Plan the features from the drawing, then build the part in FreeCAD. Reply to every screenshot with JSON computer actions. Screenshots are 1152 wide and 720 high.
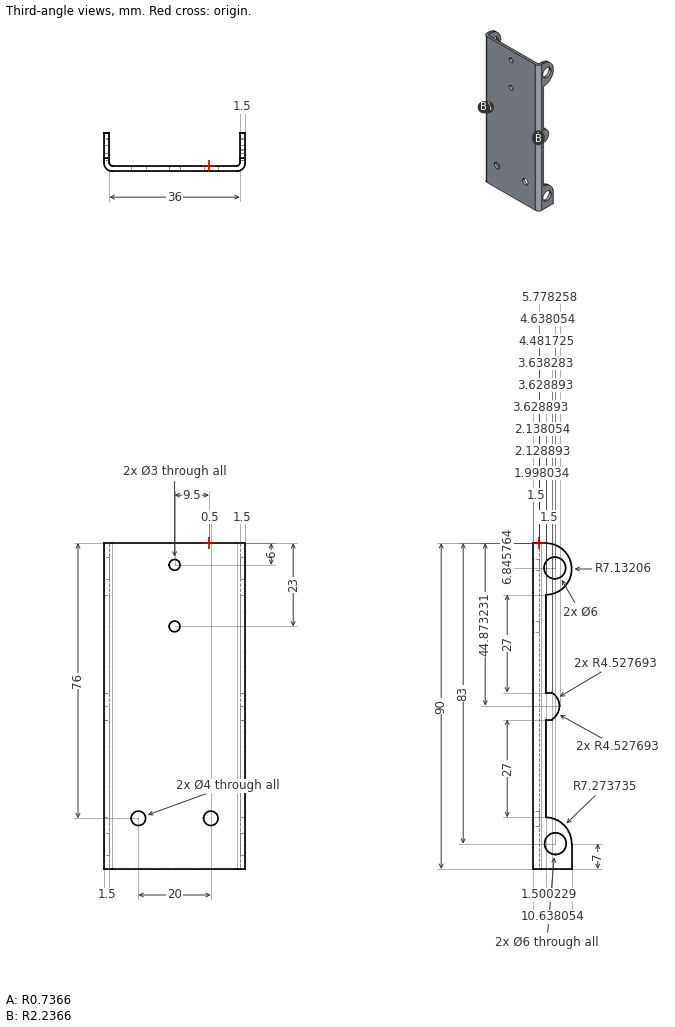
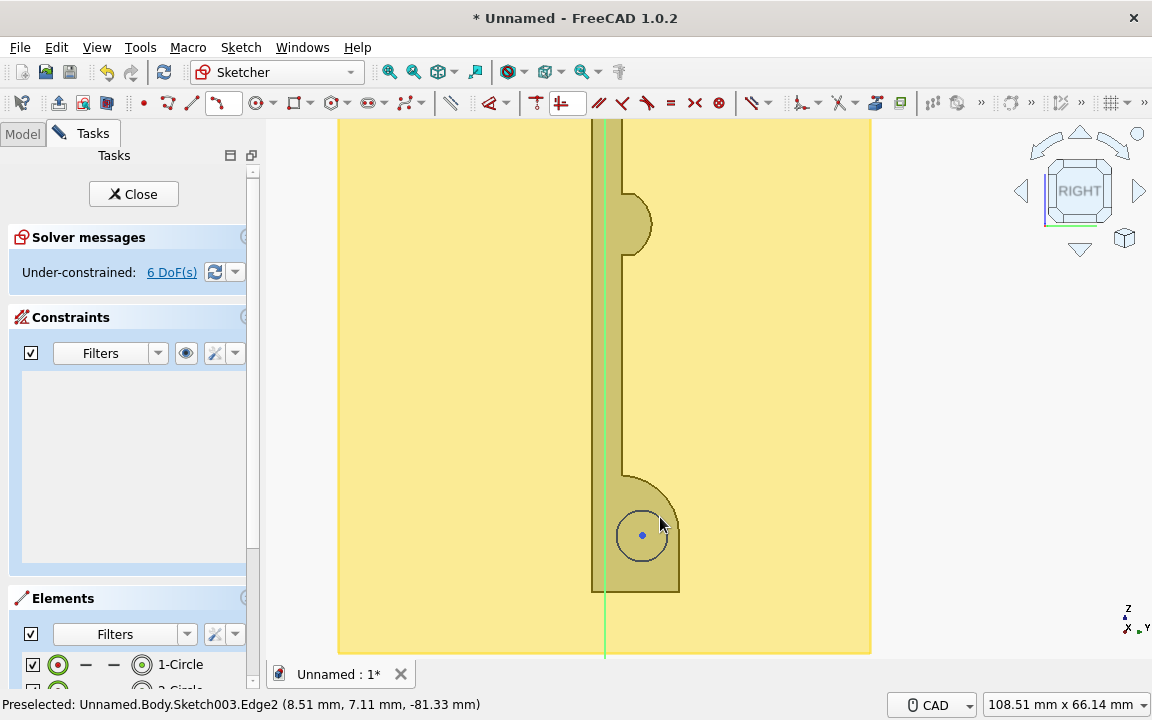
{"action": "scroll", "coordinate": [644, 537], "scroll_direction": "down", "scroll_amount": 4}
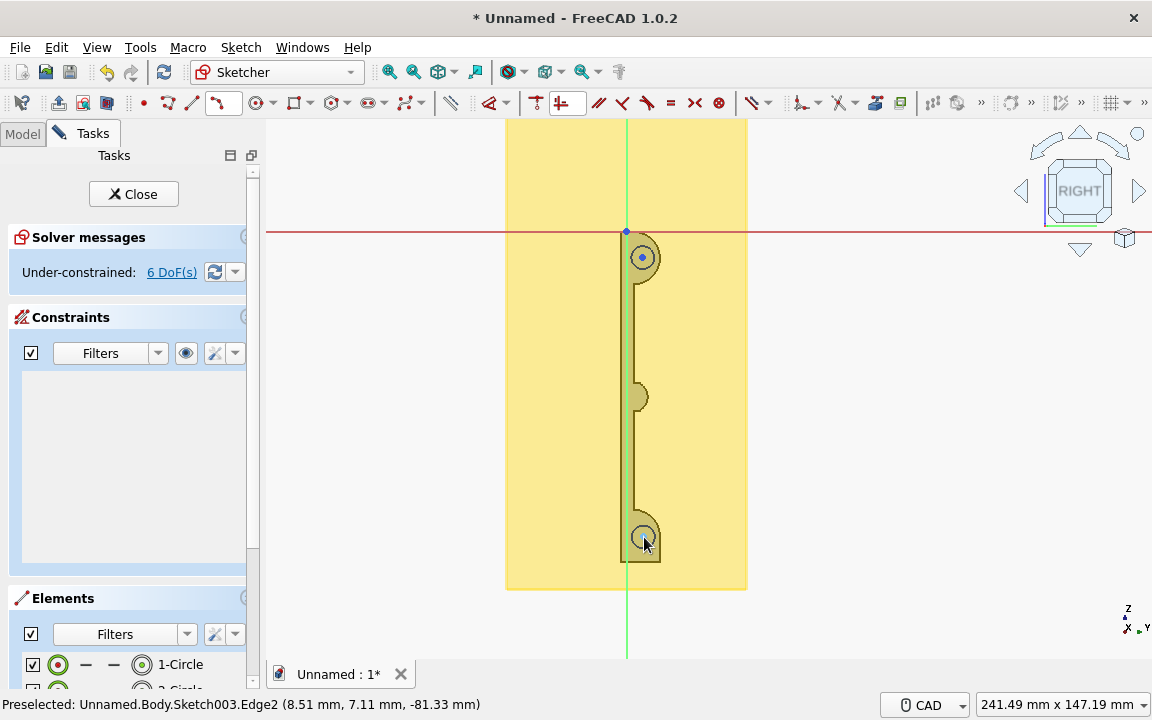
{"action": "left_click", "coordinate": [651, 249]}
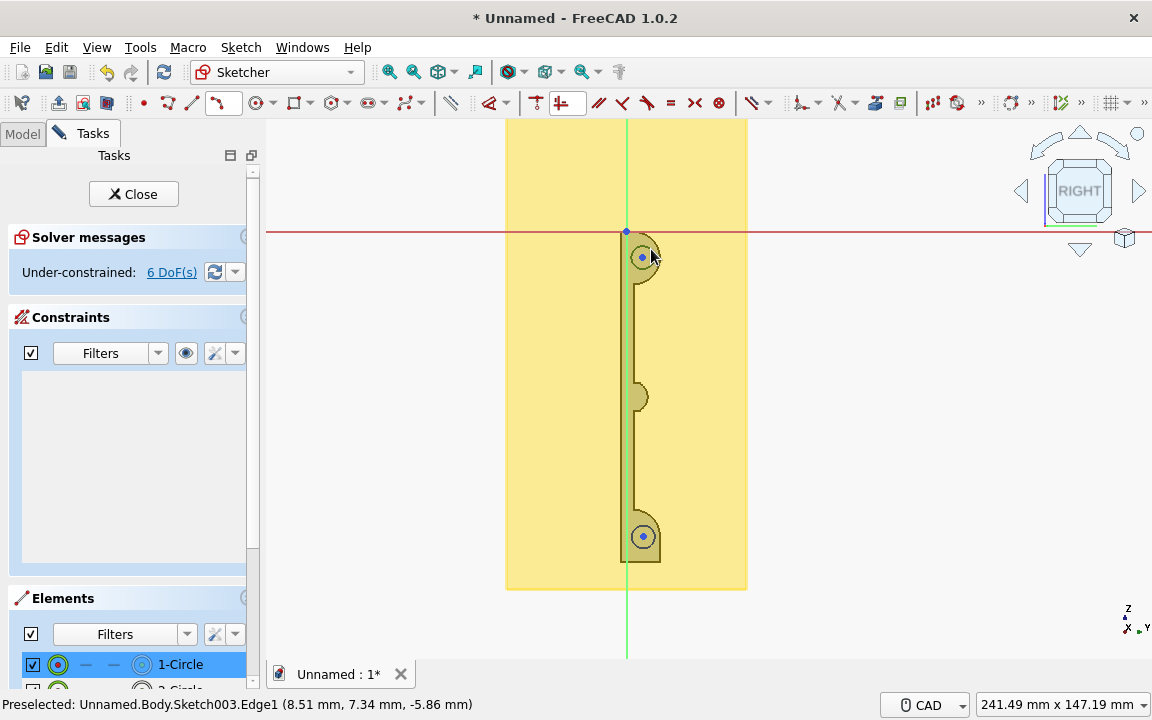
{"action": "left_click", "coordinate": [651, 529]}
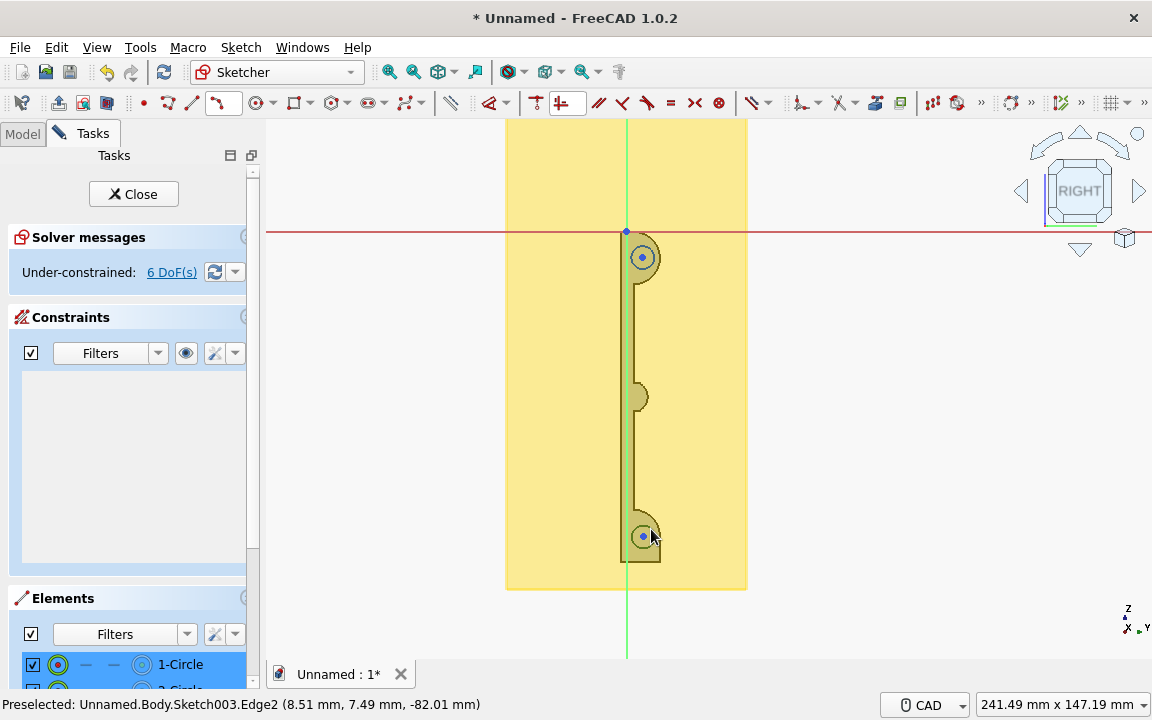
{"action": "key", "text": "e"}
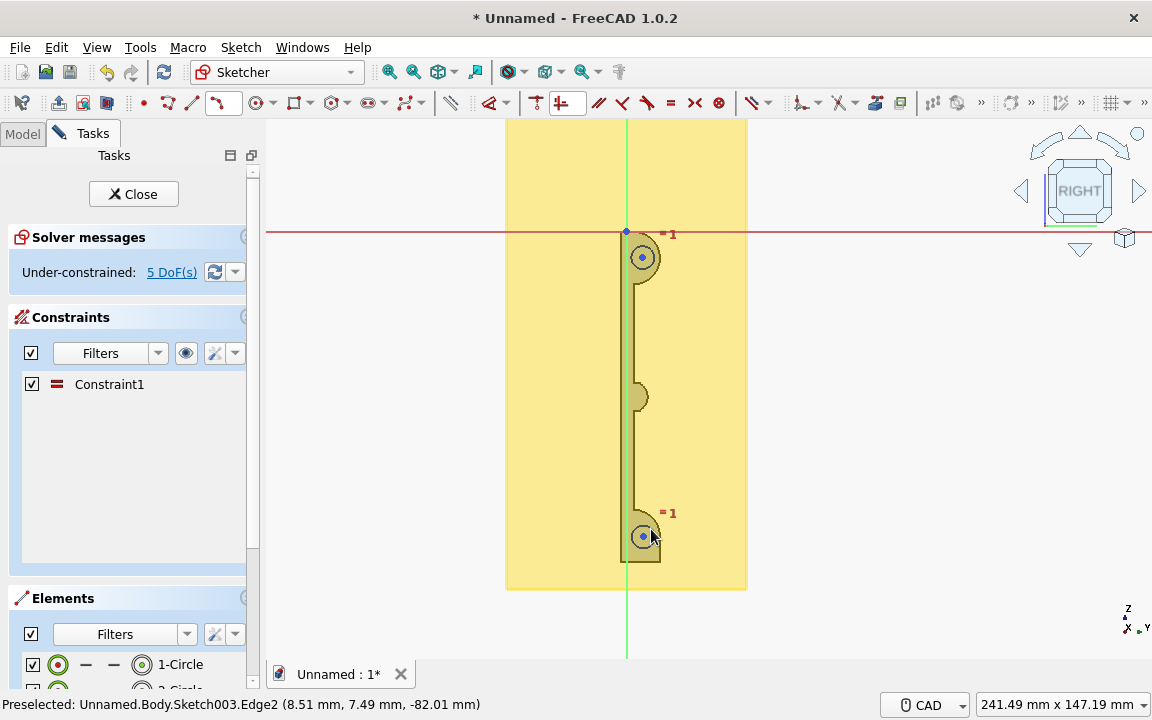
{"action": "key", "text": "d"}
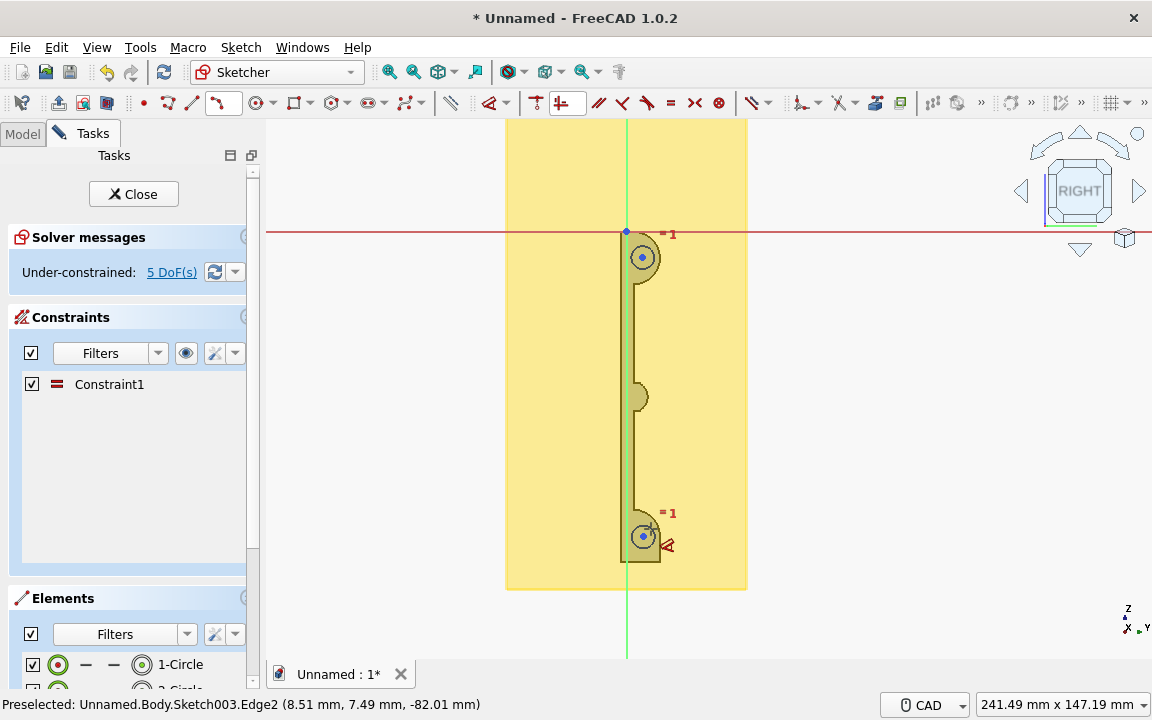
{"action": "scroll", "coordinate": [651, 249], "scroll_direction": "up", "scroll_amount": 3}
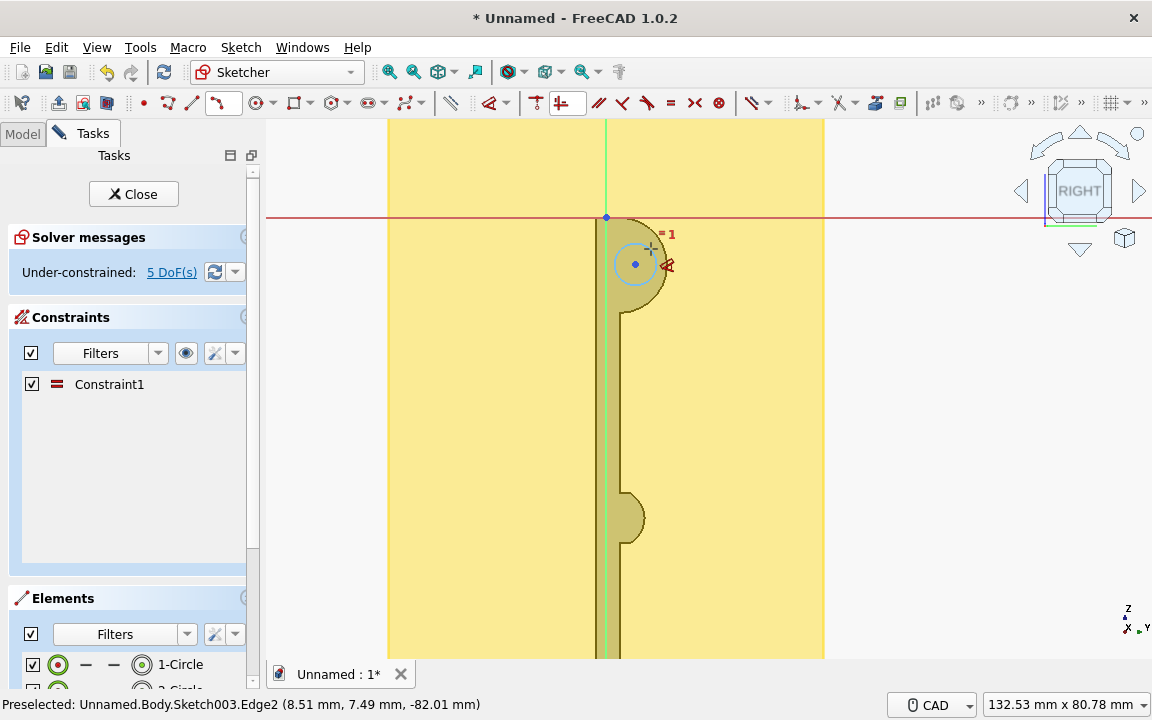
{"action": "left_click", "coordinate": [650, 250]}
{"action": "left_click", "coordinate": [686, 249]}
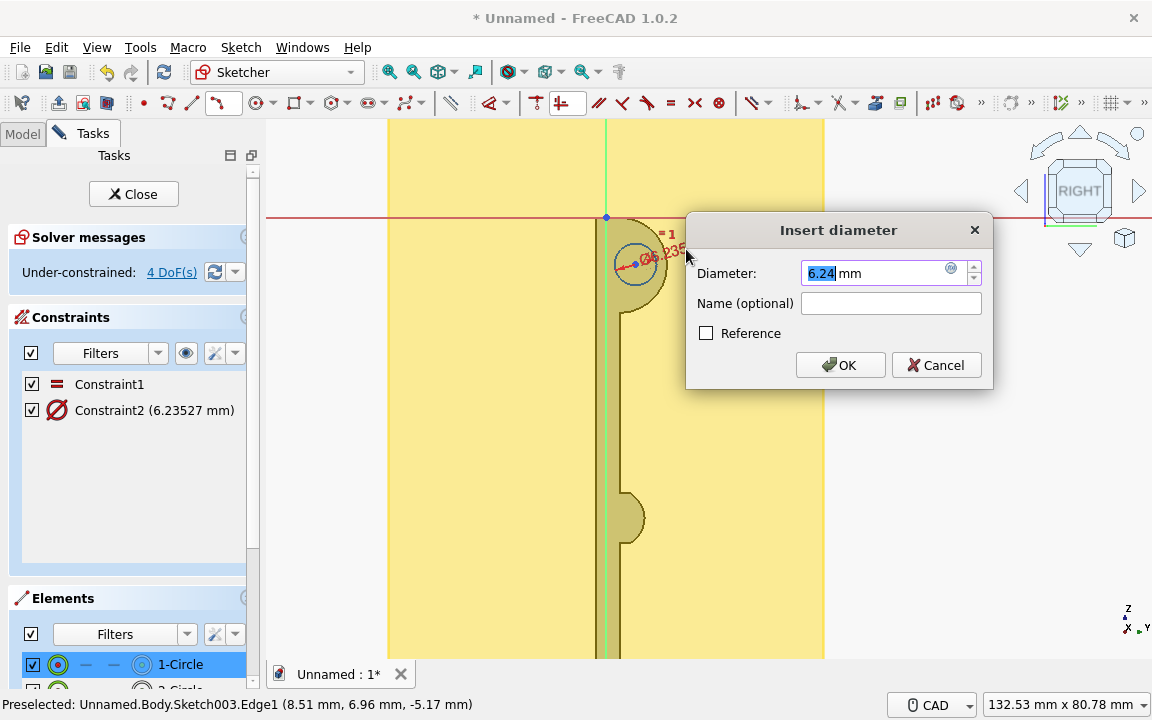
{"action": "type", "text": "6"}
{"action": "key", "text": "Return"}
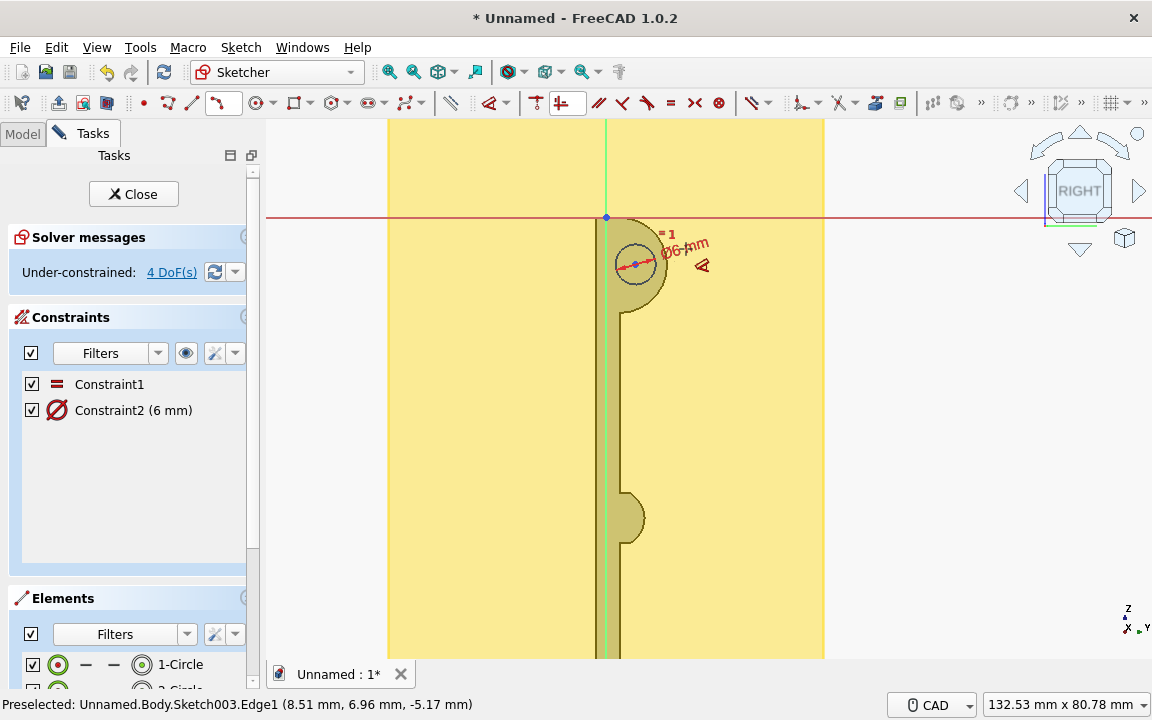
{"action": "scroll", "coordinate": [651, 248], "scroll_direction": "down", "scroll_amount": 3}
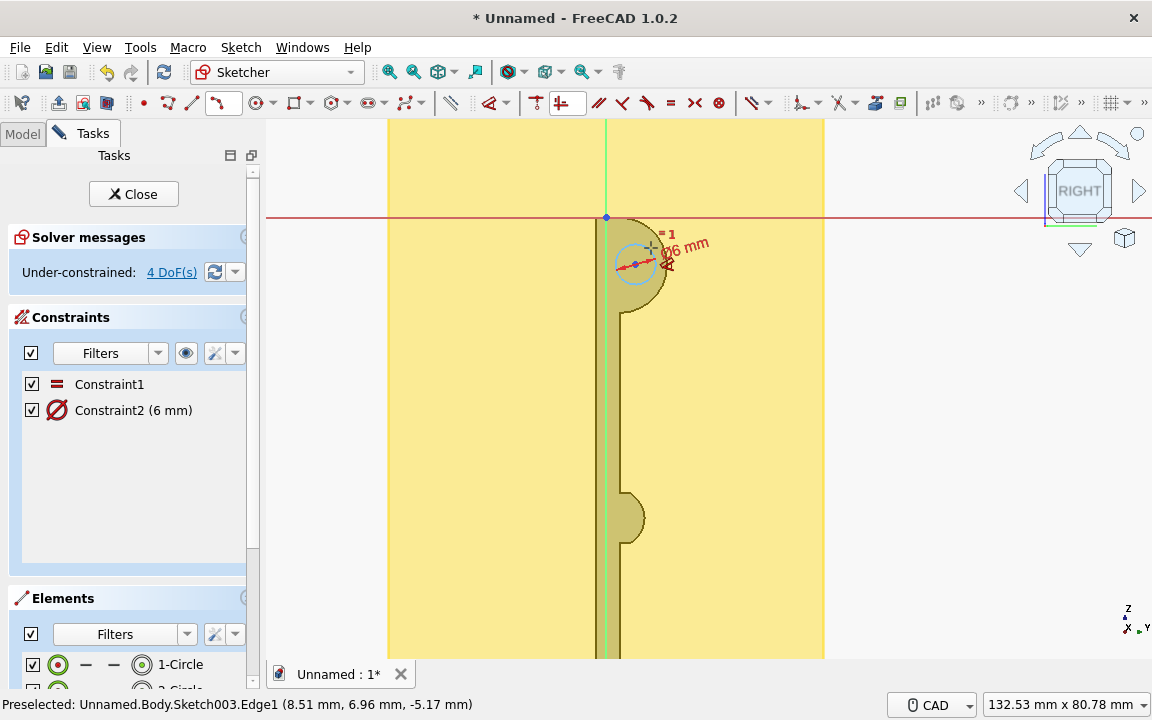
{"action": "left_click", "coordinate": [643, 537]}
{"action": "left_click", "coordinate": [593, 384]}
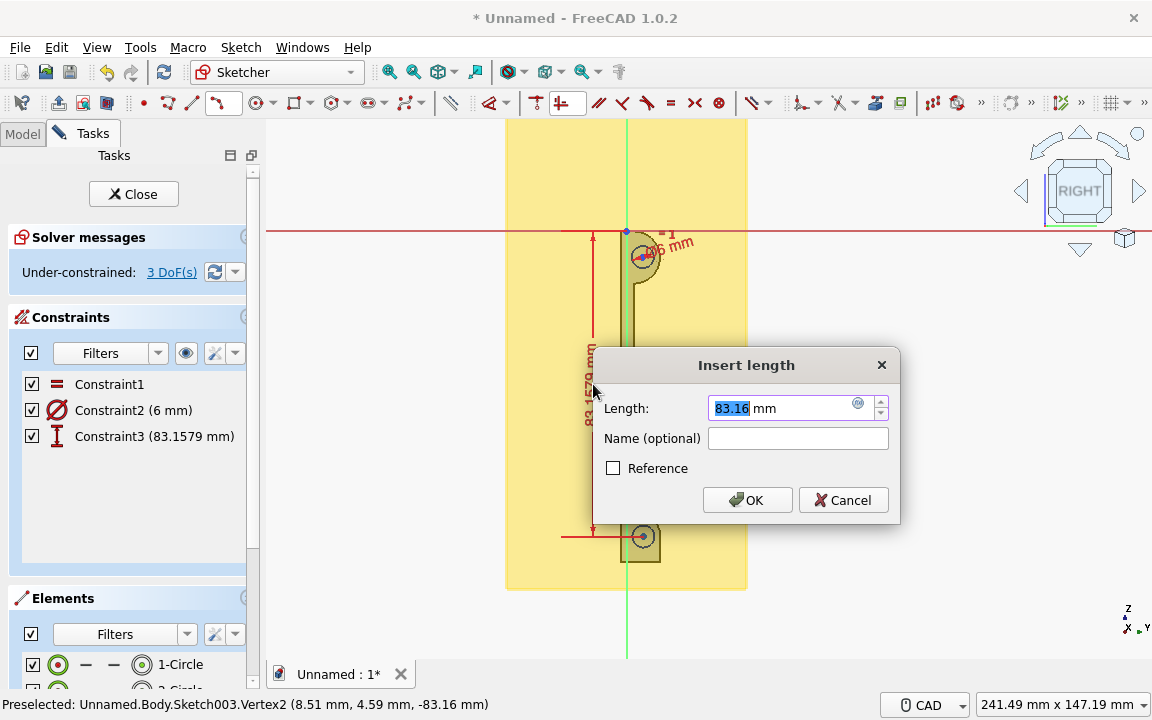
{"action": "type", "text": "83"}
{"action": "key", "text": "Return"}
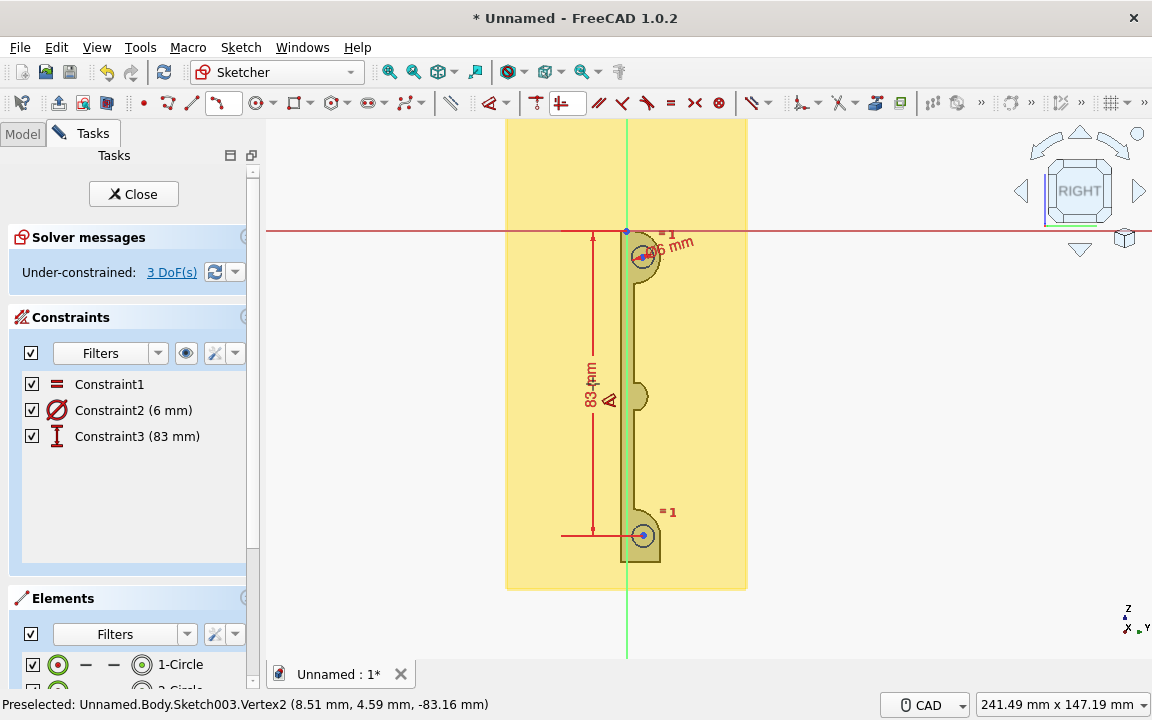
{"action": "scroll", "coordinate": [643, 257], "scroll_direction": "up", "scroll_amount": 5}